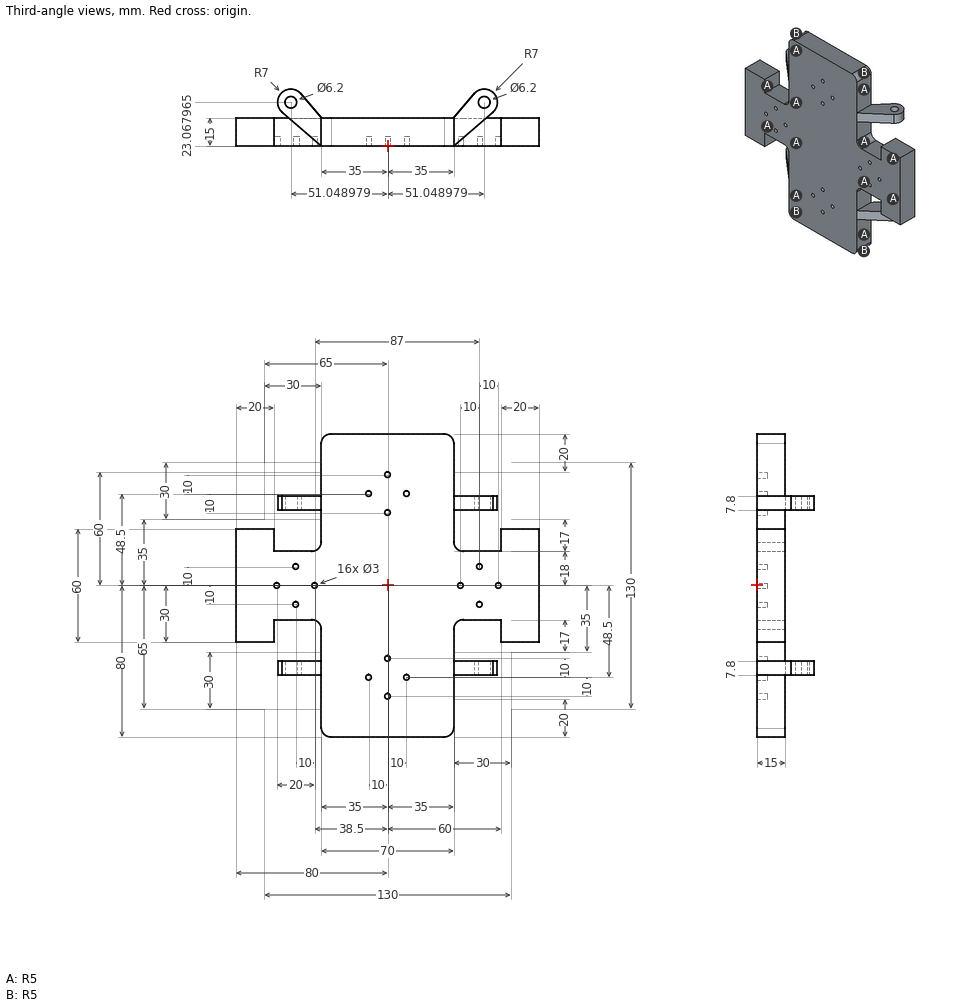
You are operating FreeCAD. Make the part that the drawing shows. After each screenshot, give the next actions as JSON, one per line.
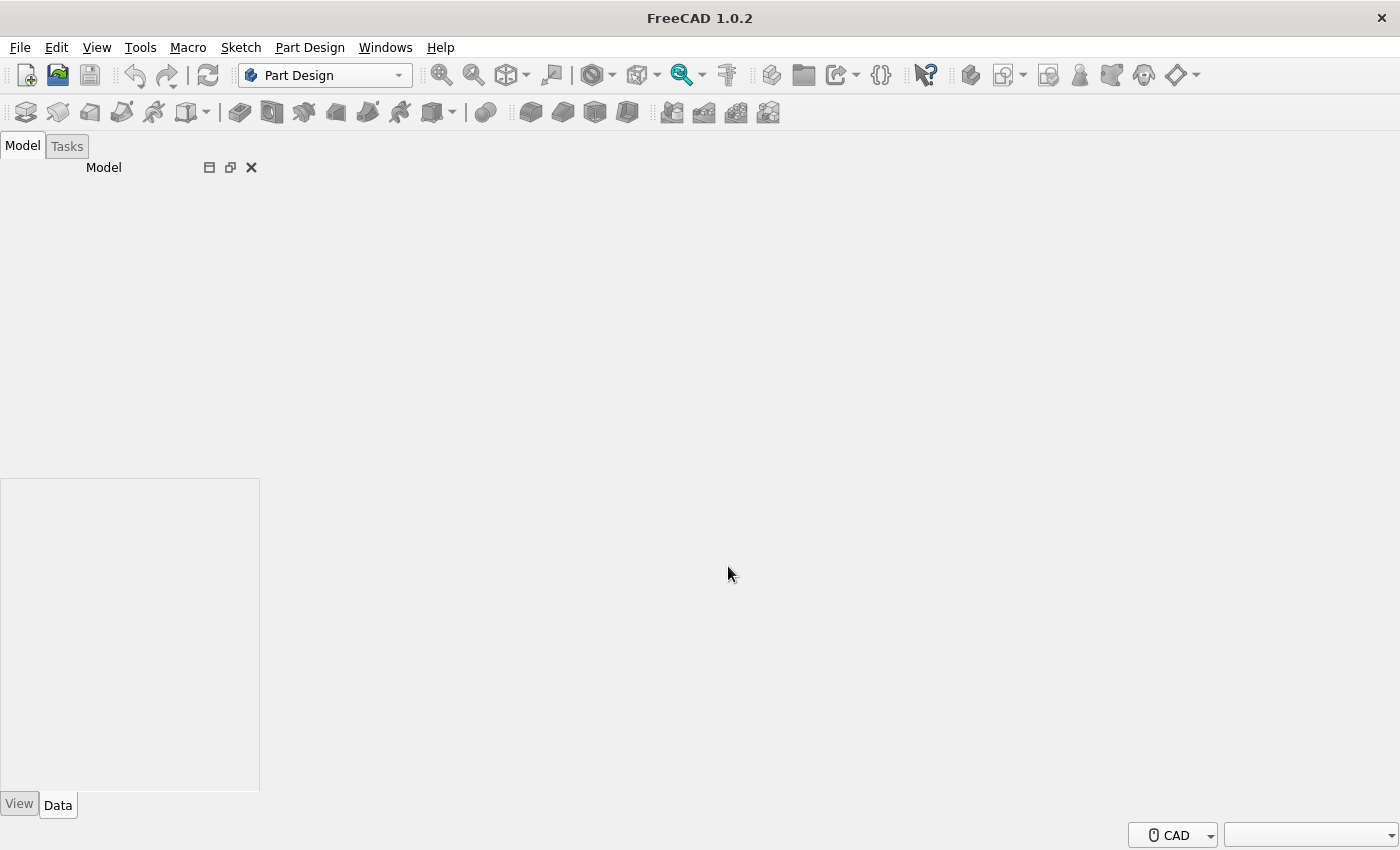
{"action": "left_click", "coordinate": [26, 76]}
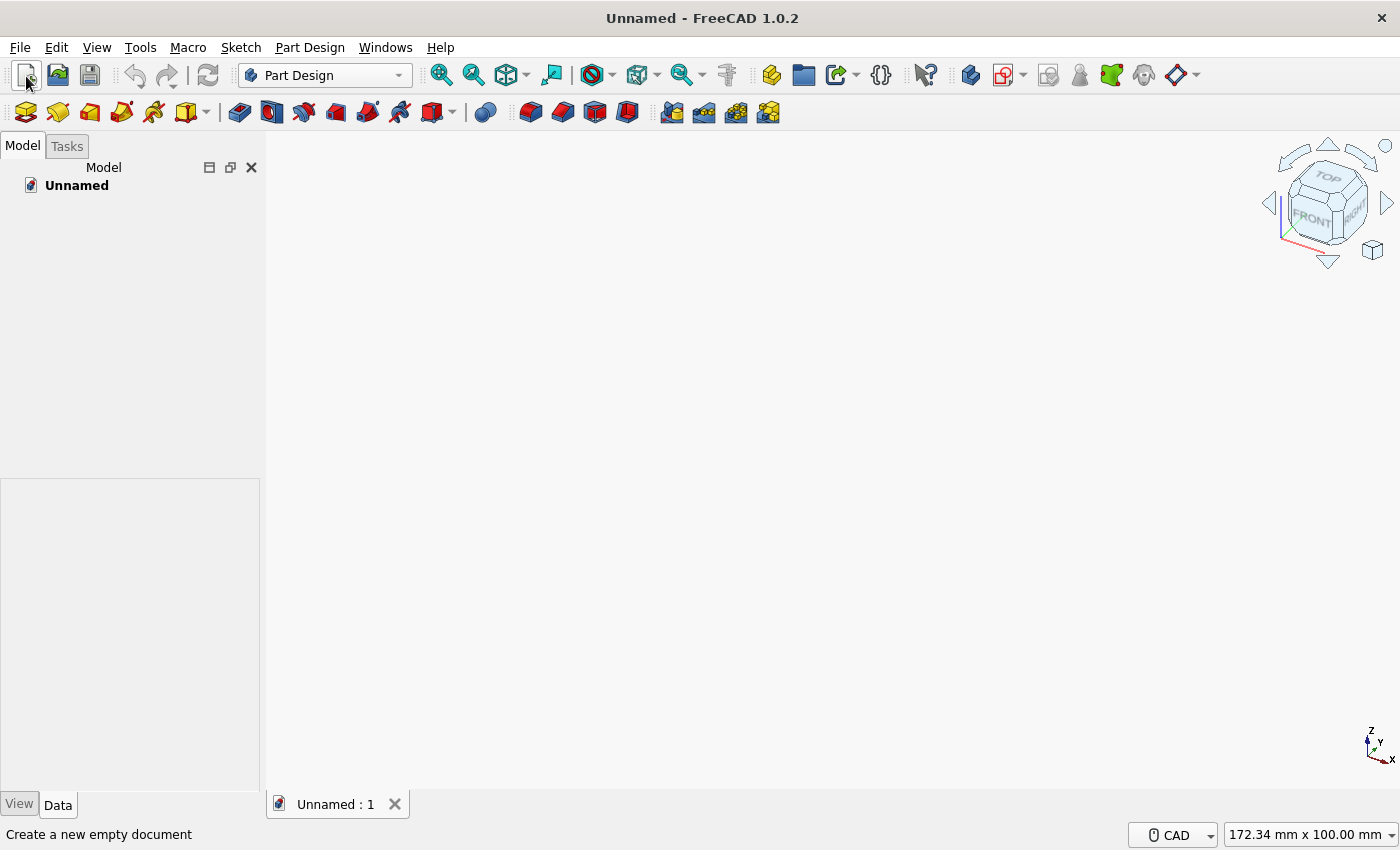
{"action": "left_click", "coordinate": [1004, 76]}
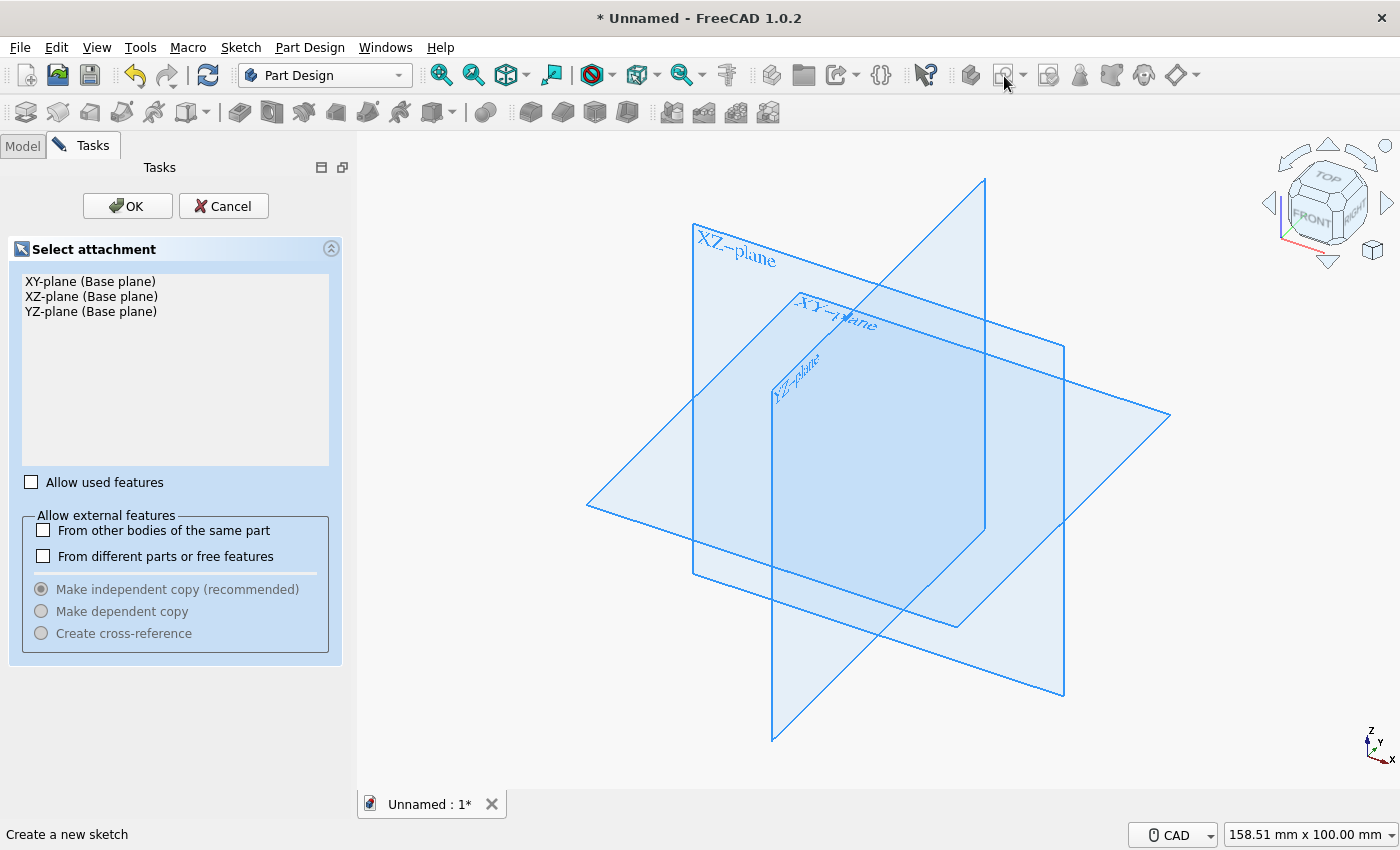
{"action": "left_click", "coordinate": [82, 296]}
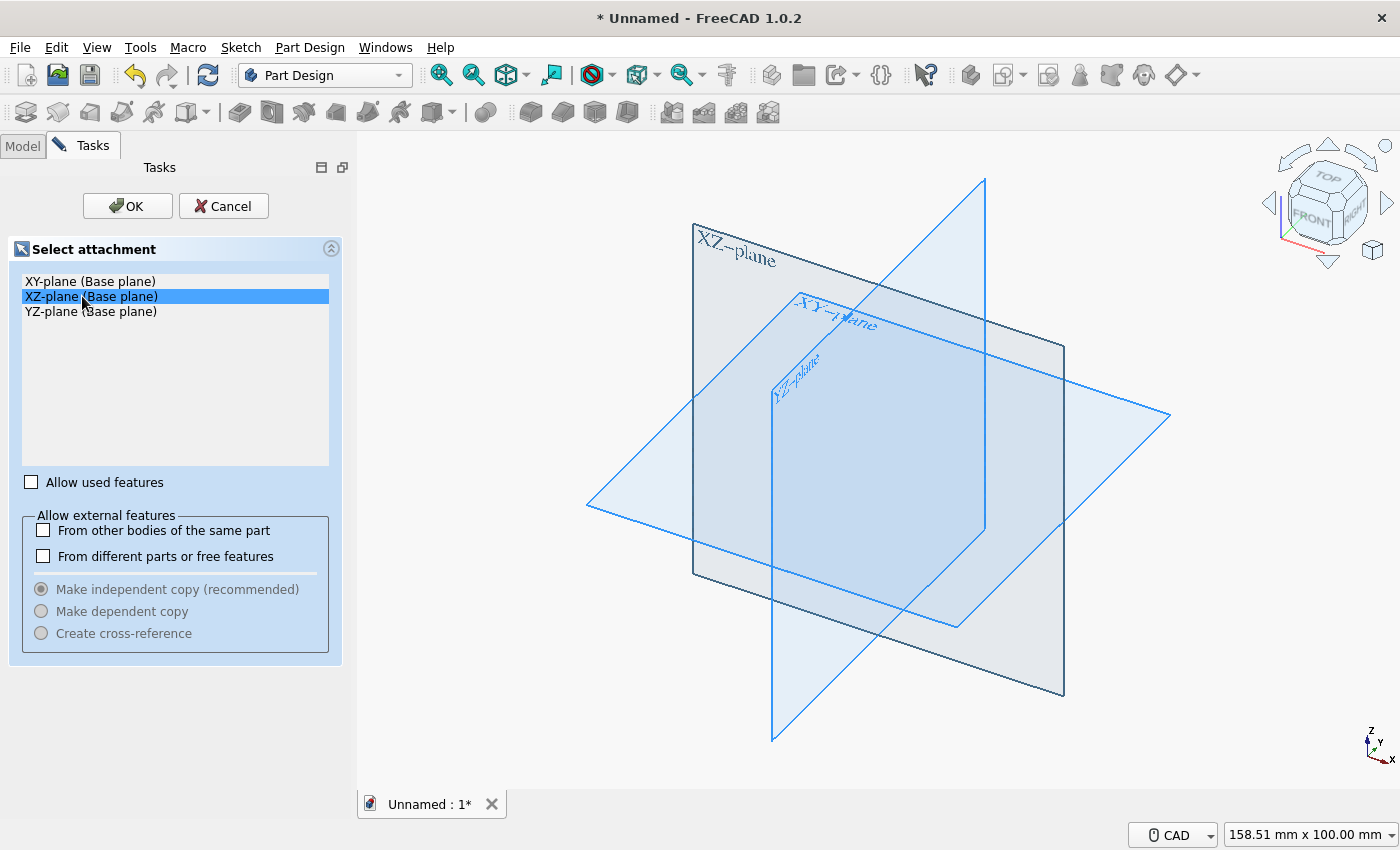
{"action": "left_click", "coordinate": [128, 206]}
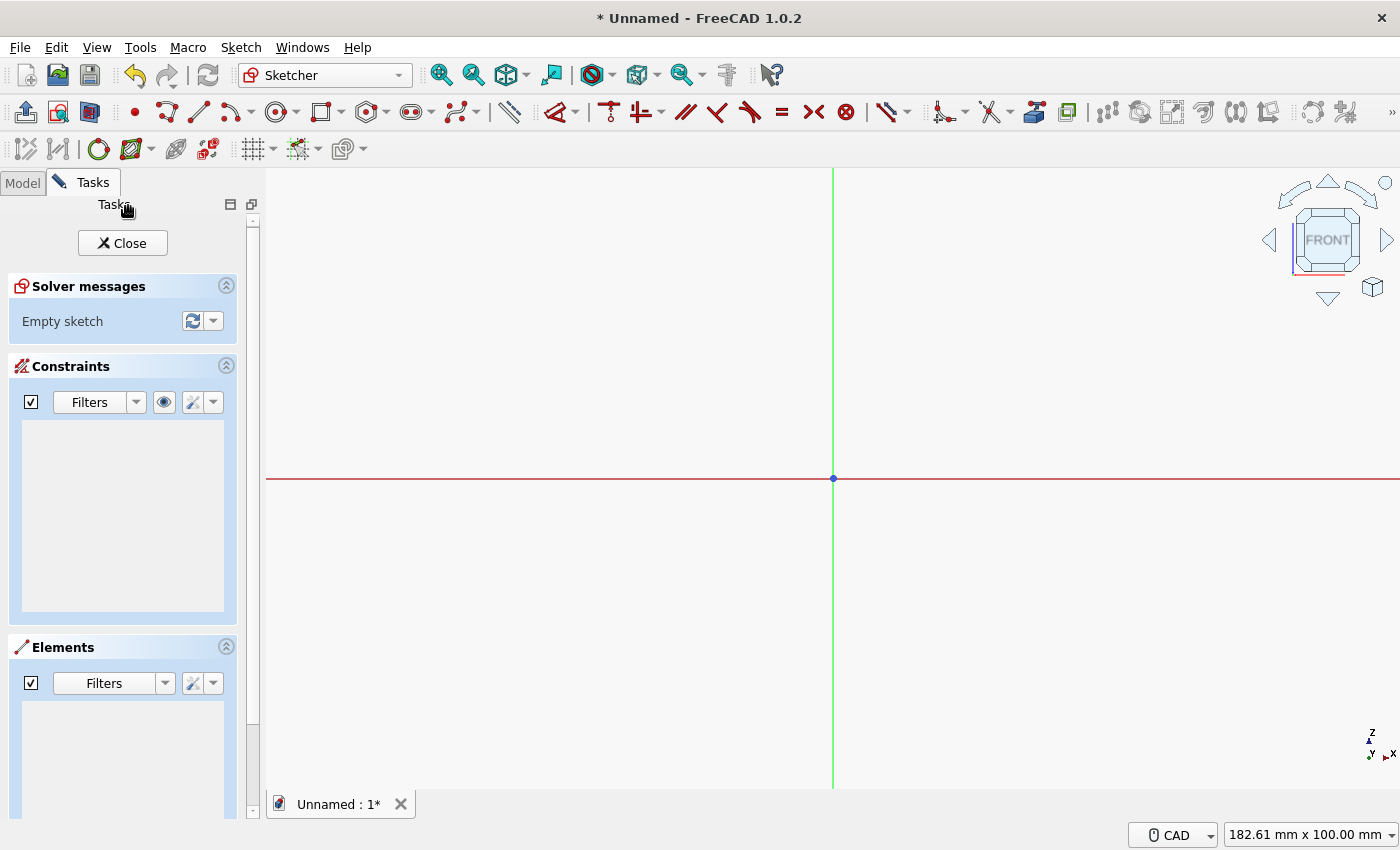
{"action": "scroll", "coordinate": [709, 478], "scroll_direction": "down", "scroll_amount": 4}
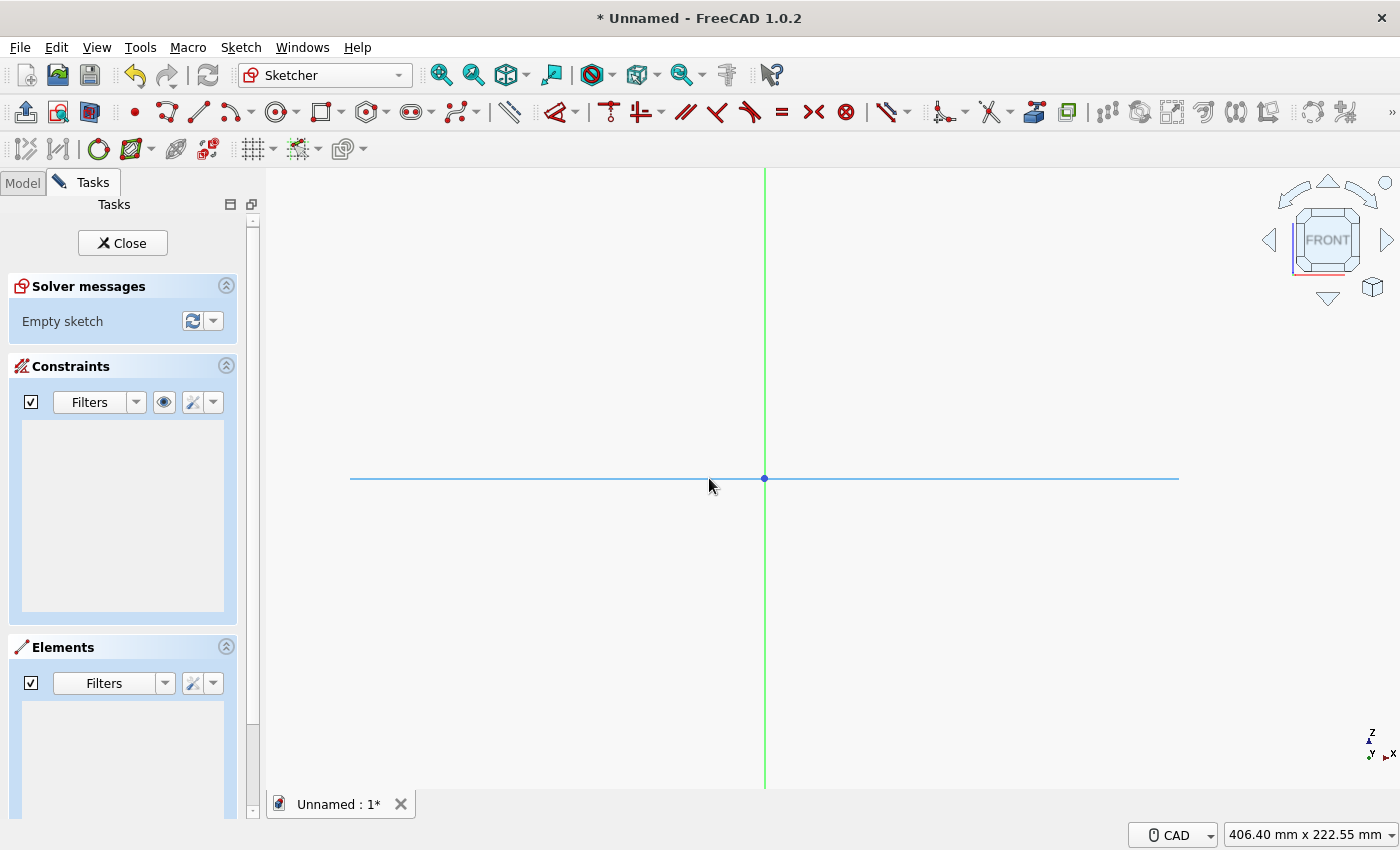
{"action": "left_click", "coordinate": [344, 112]}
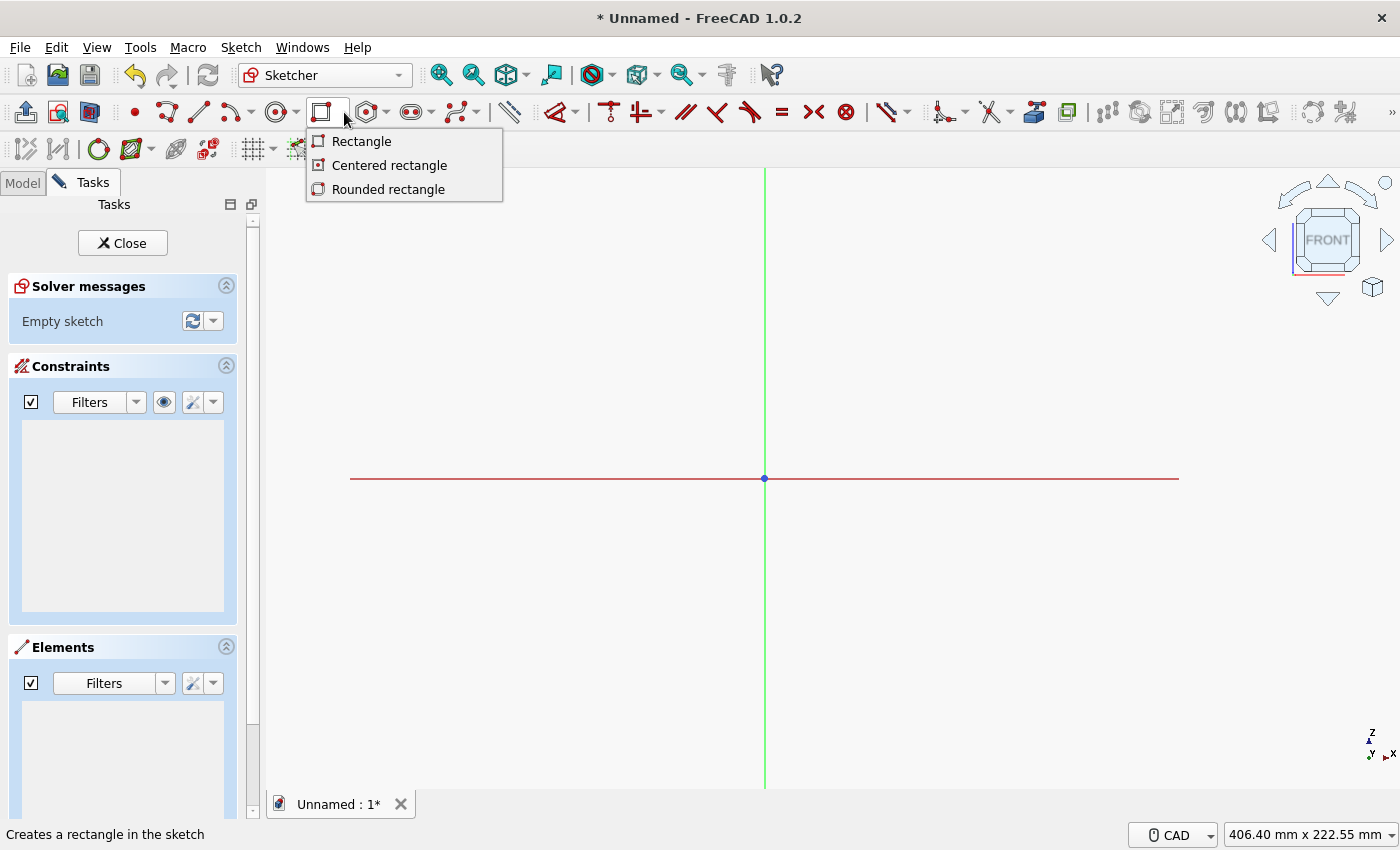
{"action": "left_click", "coordinate": [404, 165]}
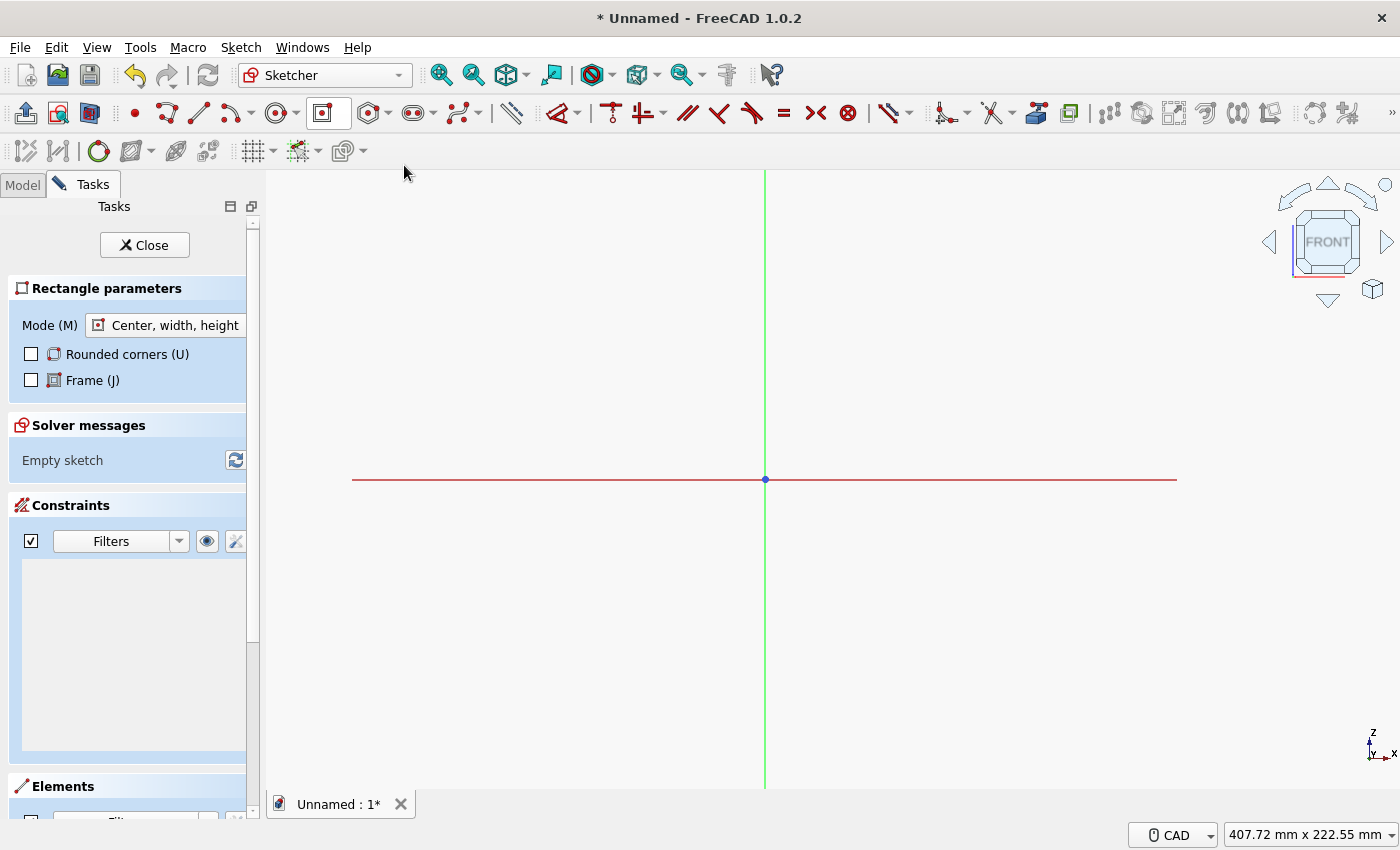
{"action": "left_click", "coordinate": [765, 480]}
{"action": "mouse_move", "coordinate": [946, 299]}